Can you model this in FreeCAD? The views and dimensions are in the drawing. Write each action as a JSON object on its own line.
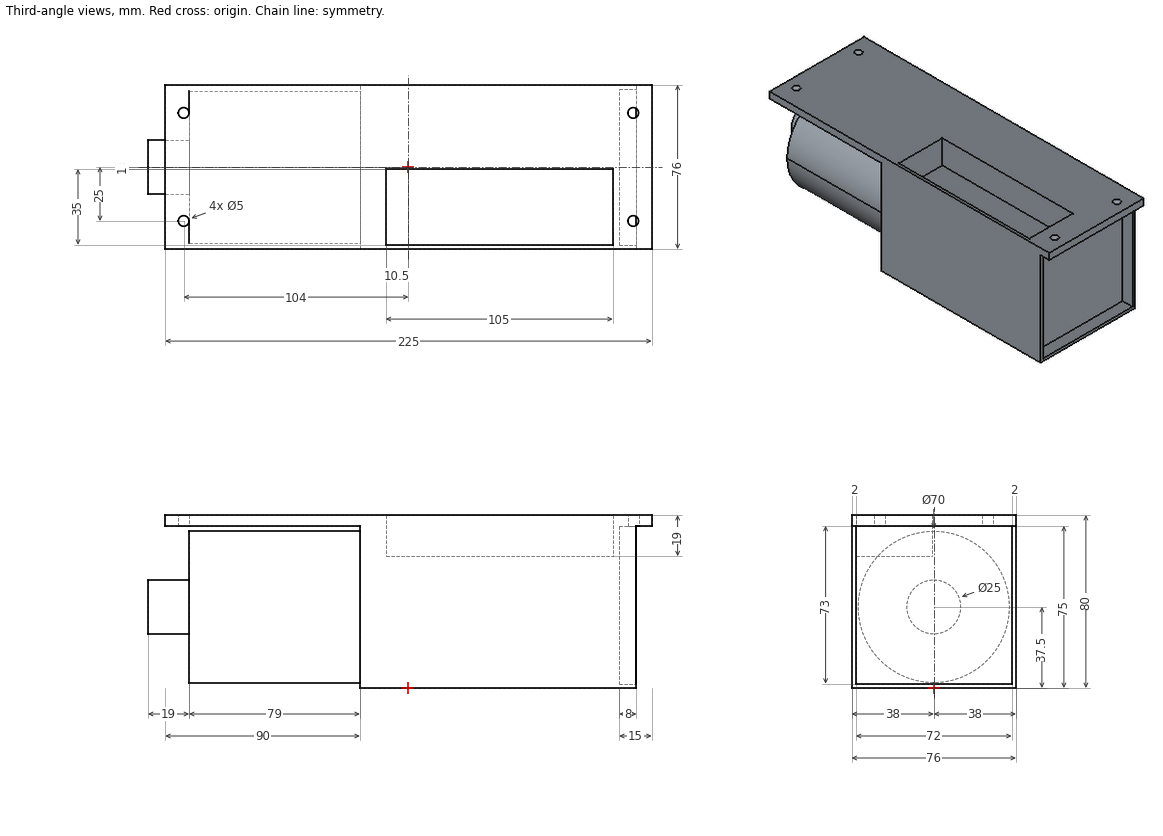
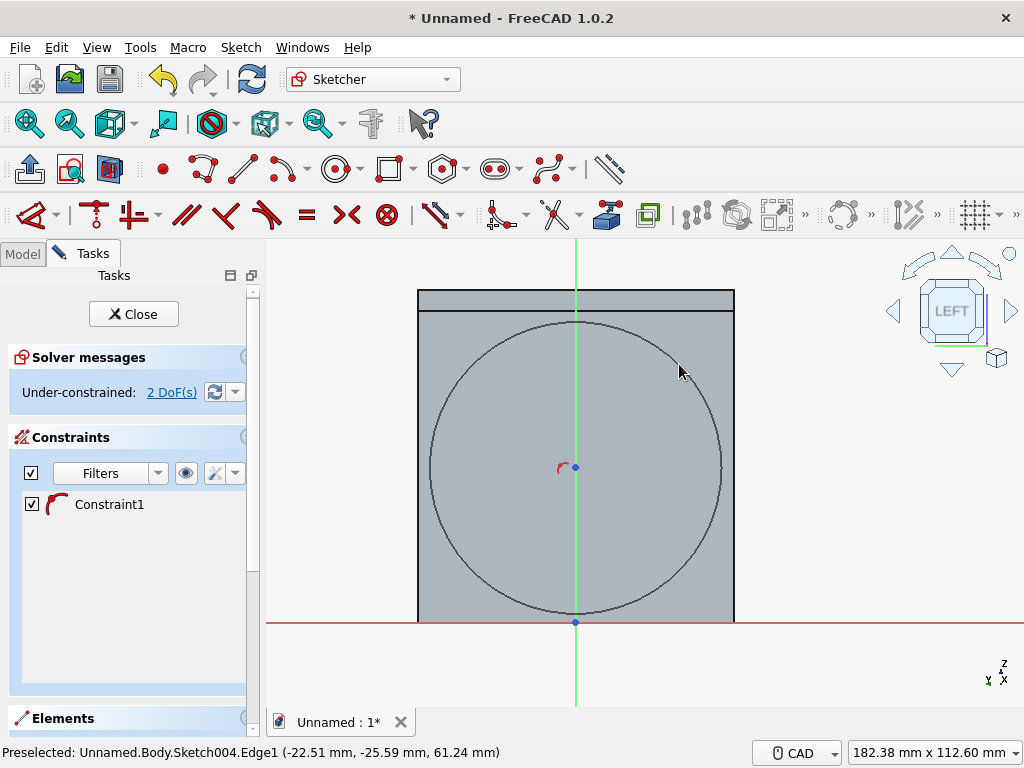
{"action": "key", "text": "d"}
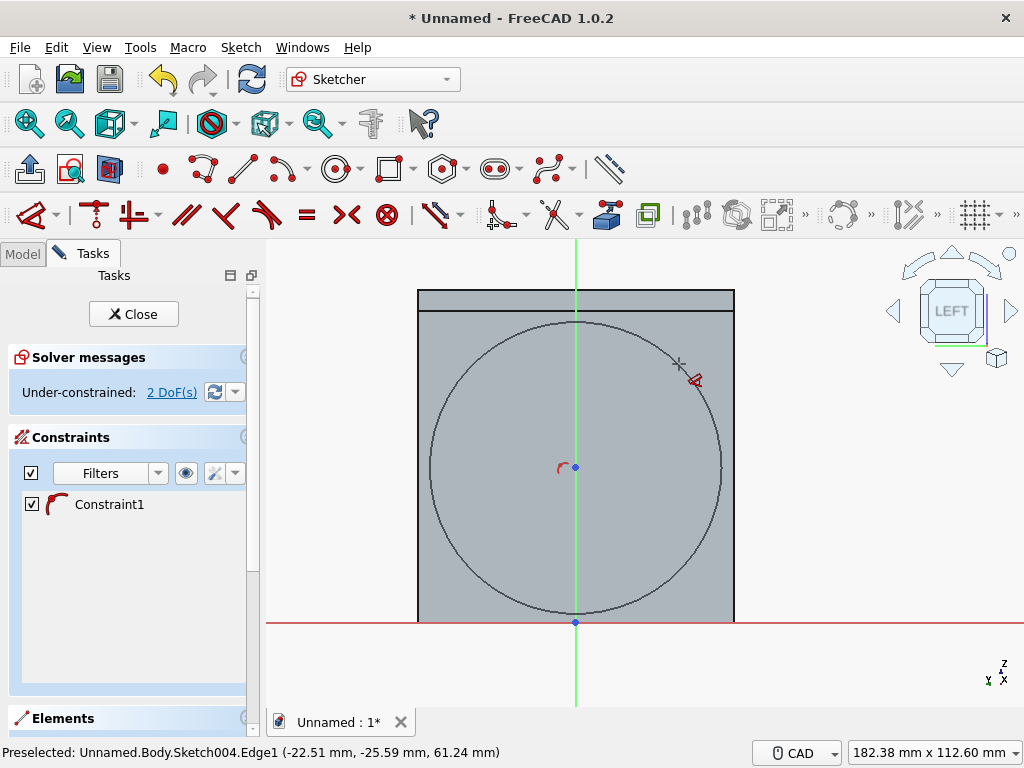
{"action": "left_click", "coordinate": [679, 365]}
{"action": "left_click", "coordinate": [702, 342]}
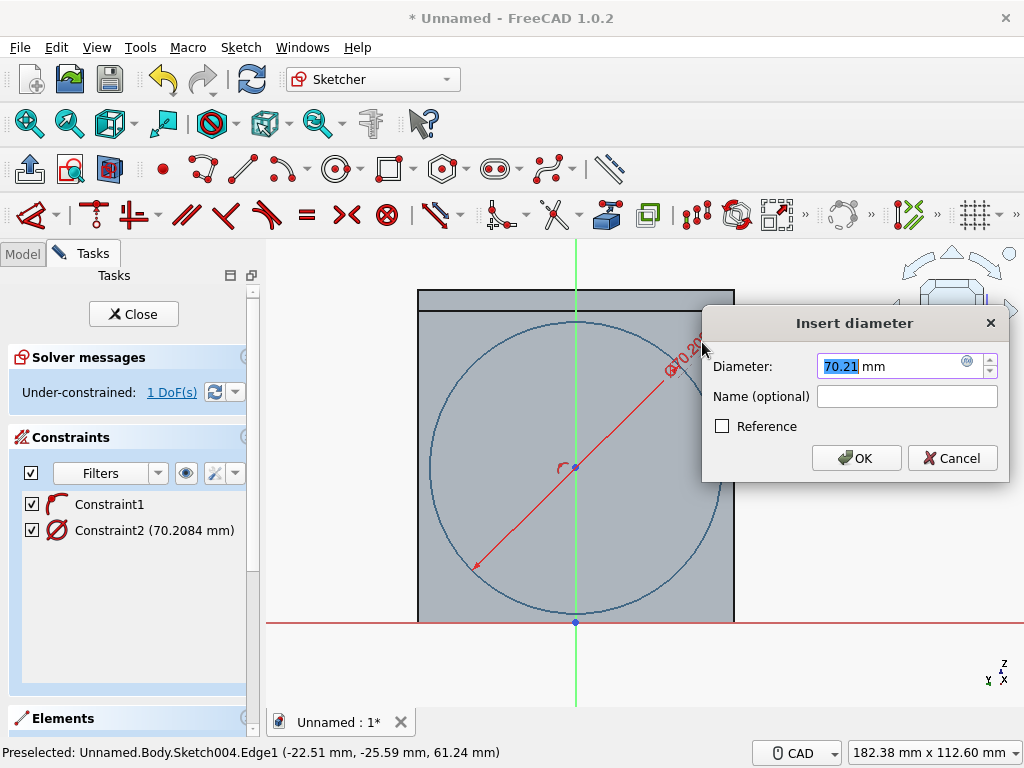
{"action": "type", "text": "70"}
{"action": "key", "text": "Return"}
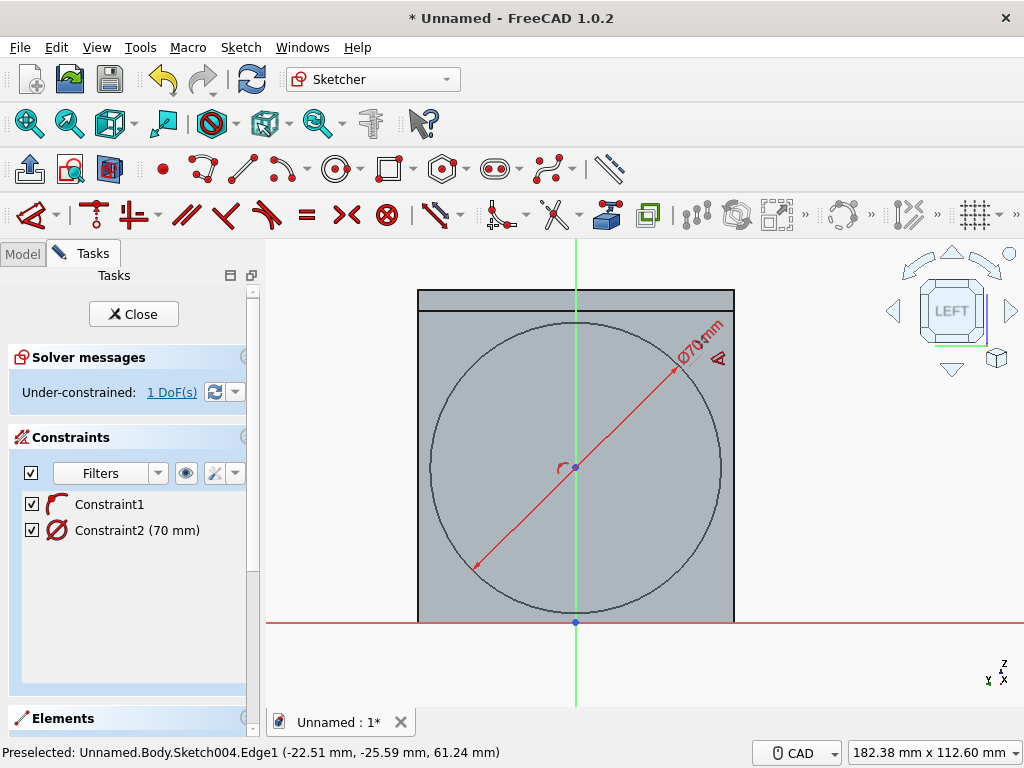
{"action": "left_click", "coordinate": [576, 468]}
{"action": "left_click", "coordinate": [610, 545]}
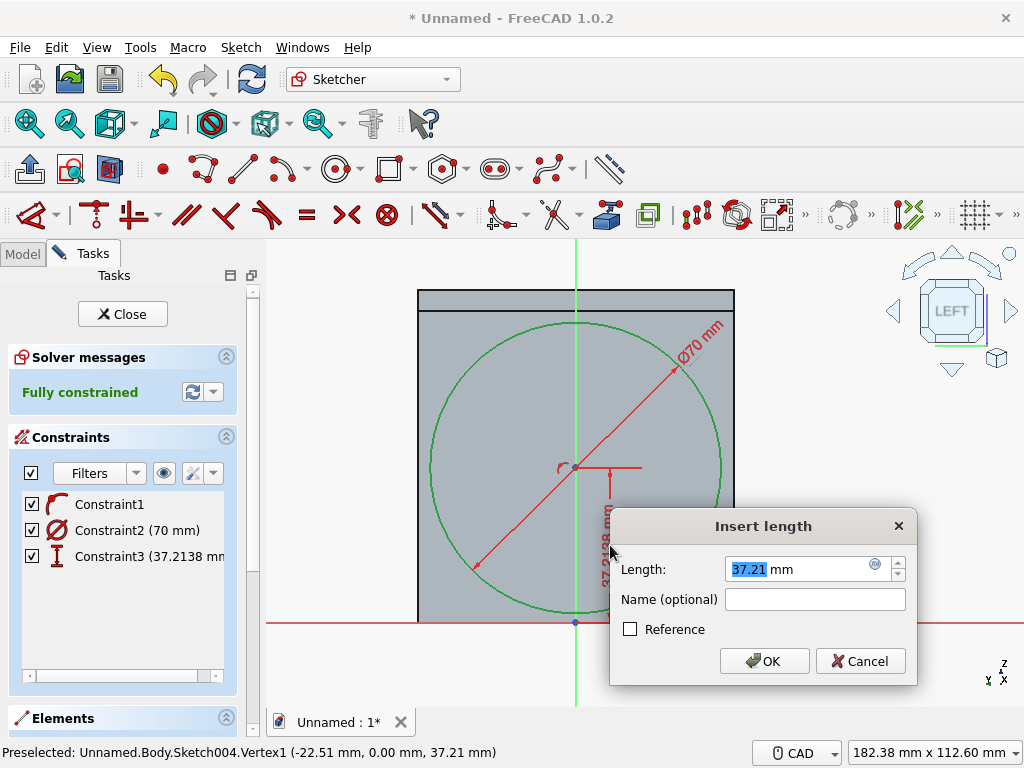
{"action": "type", "text": "37.5"}
{"action": "key", "text": "Return"}
{"action": "key", "text": "Escape"}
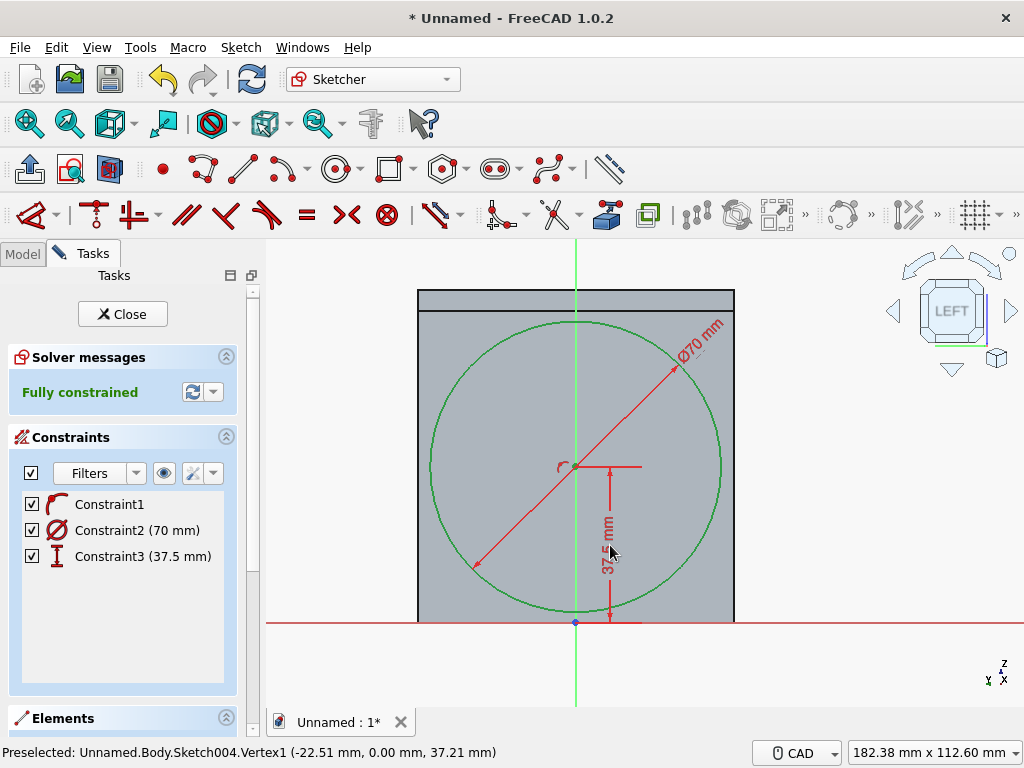
{"action": "left_click", "coordinate": [123, 314]}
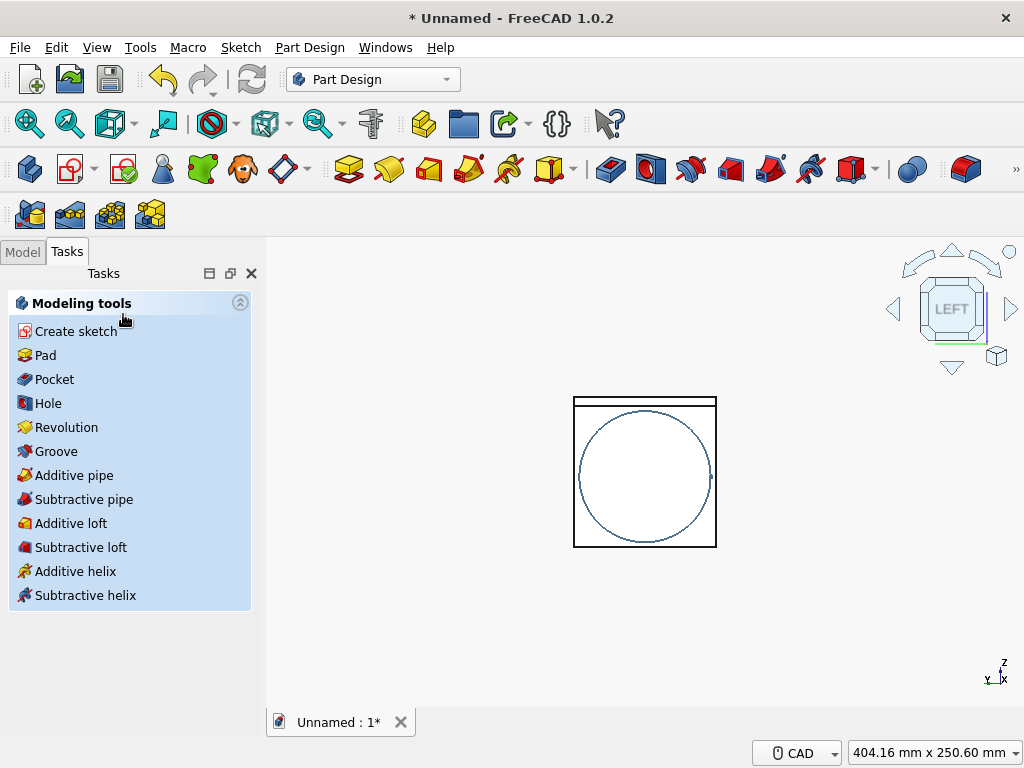
{"action": "left_click", "coordinate": [350, 170]}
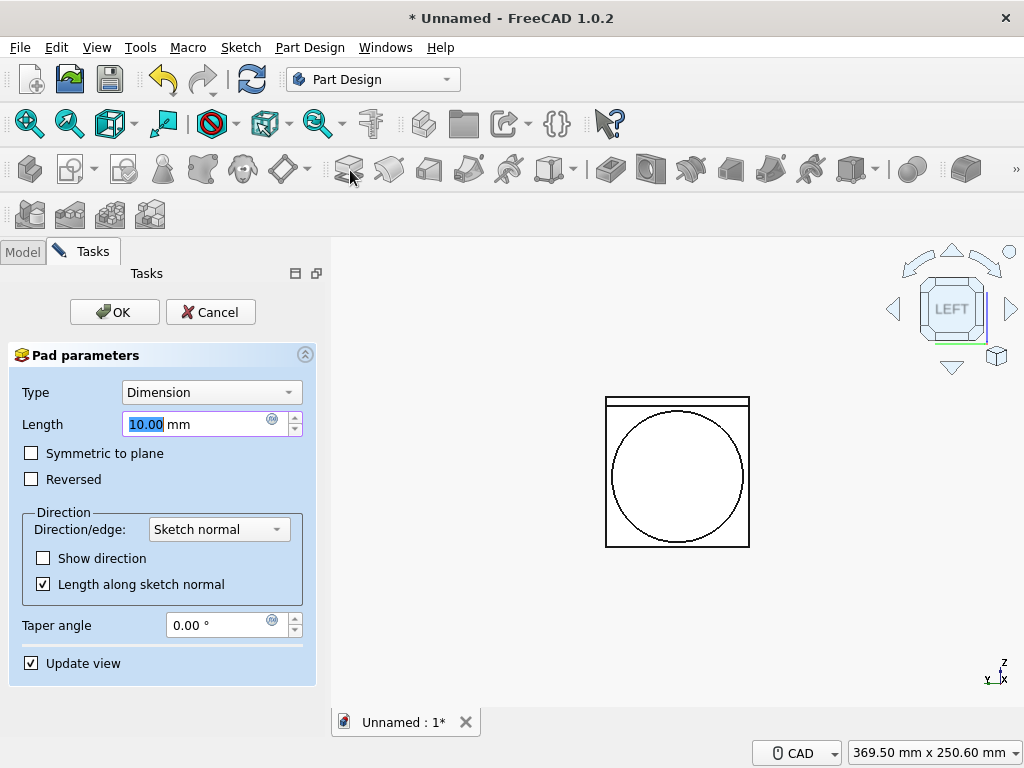
{"action": "type", "text": "79"}
{"action": "key", "text": "Tab"}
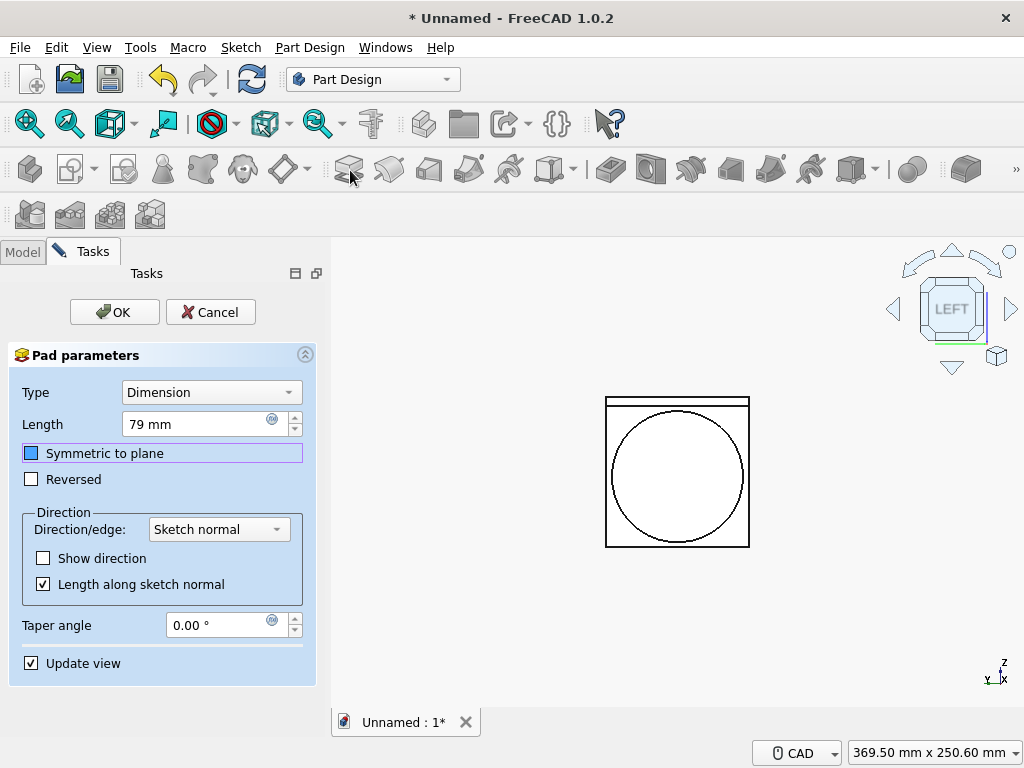
{"action": "left_click", "coordinate": [115, 312]}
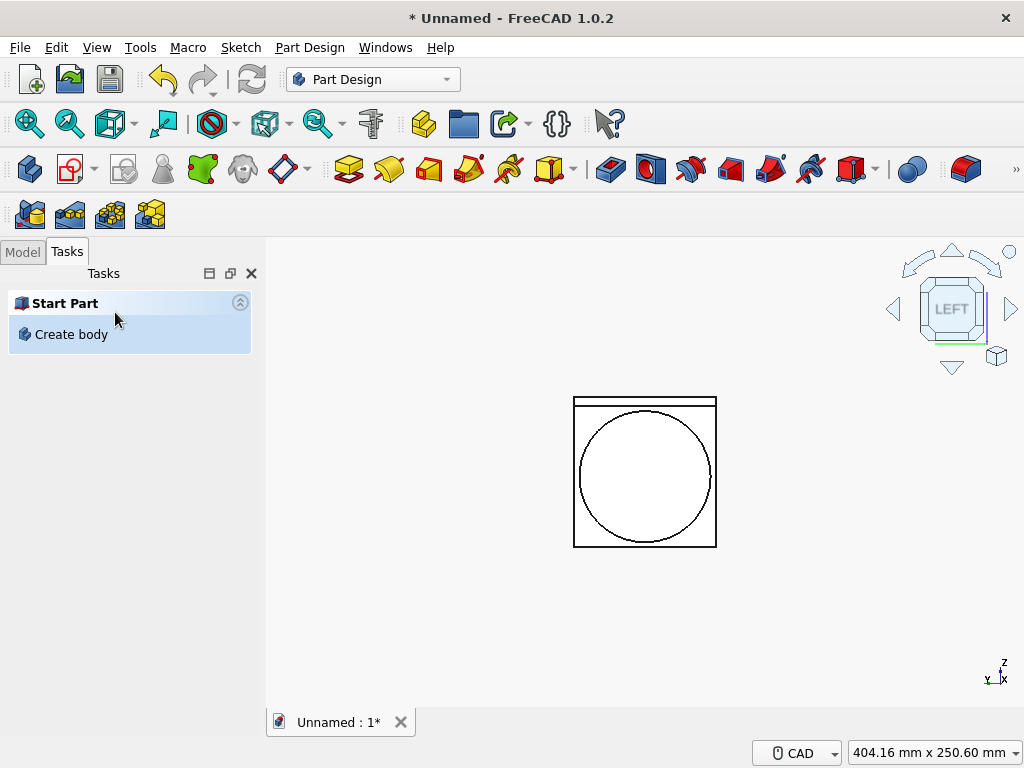
{"action": "key", "text": "v f"}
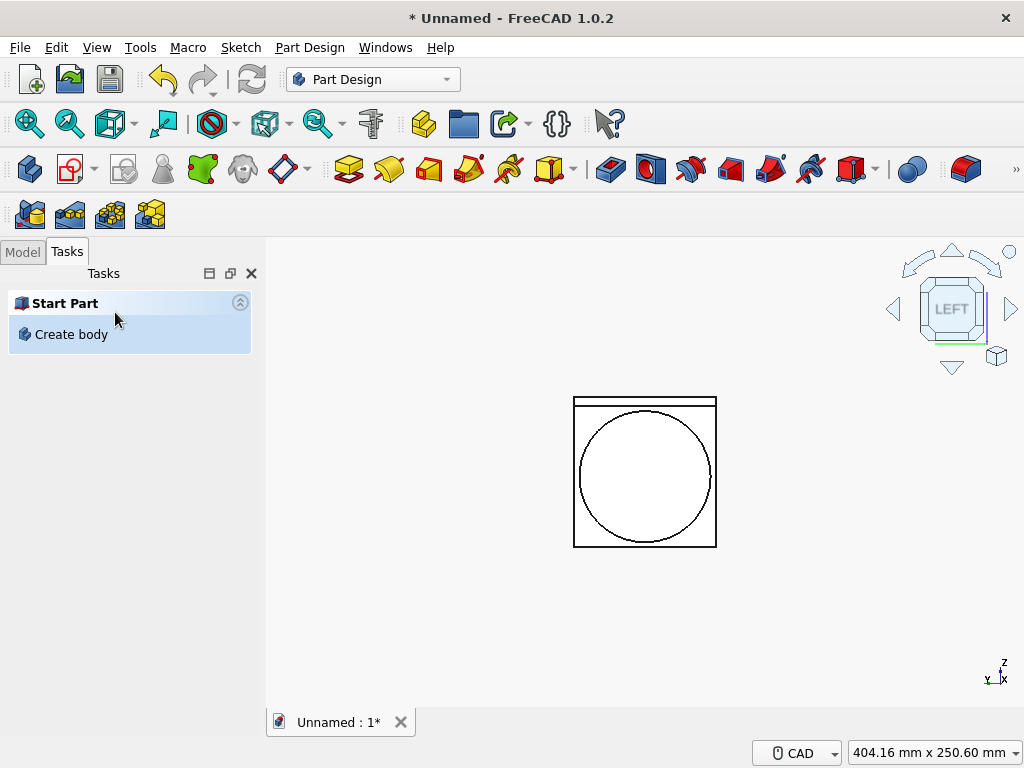
{"action": "left_click", "coordinate": [645, 476]}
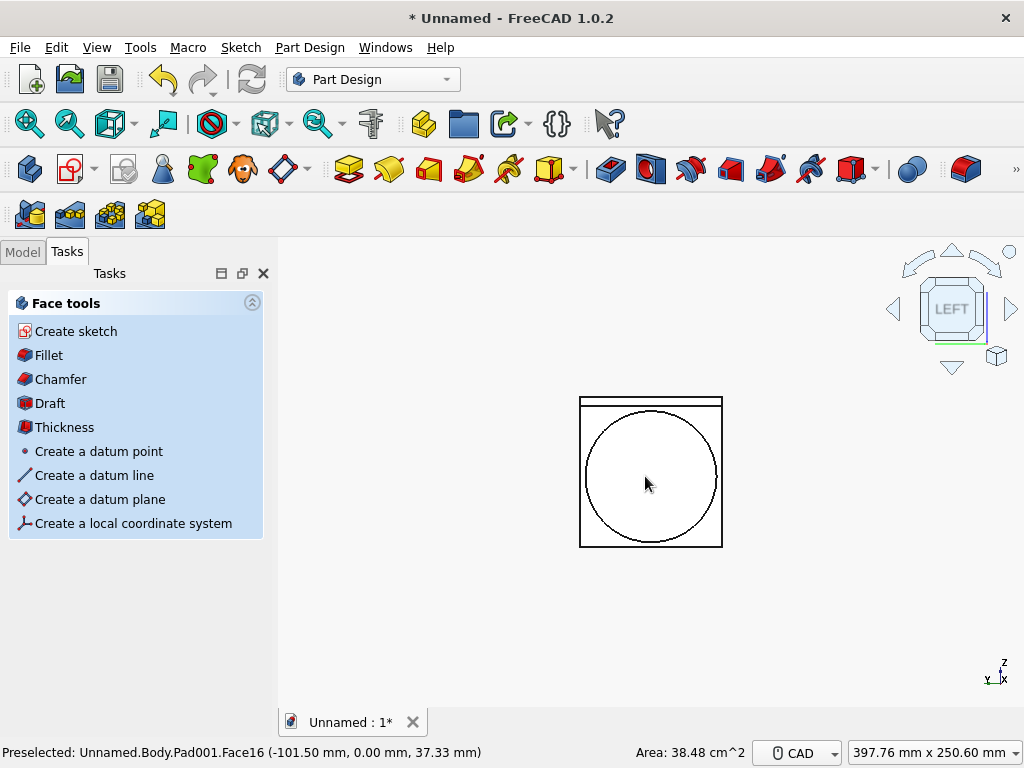
{"action": "left_click", "coordinate": [70, 170]}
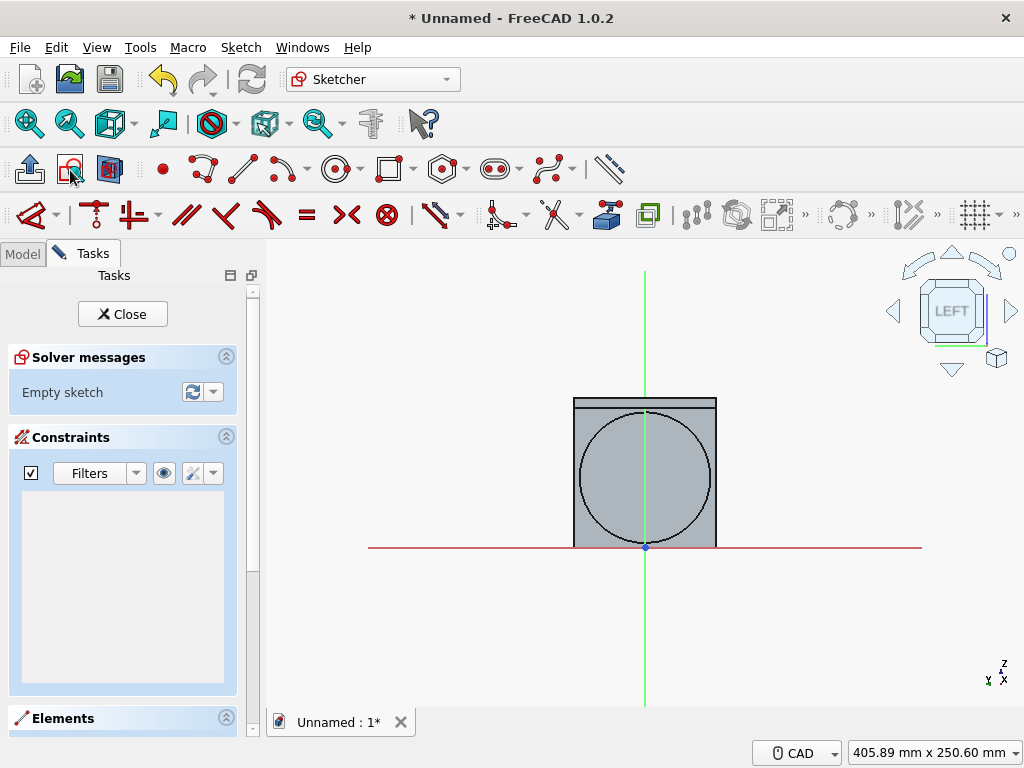
{"action": "key", "text": "q s"}